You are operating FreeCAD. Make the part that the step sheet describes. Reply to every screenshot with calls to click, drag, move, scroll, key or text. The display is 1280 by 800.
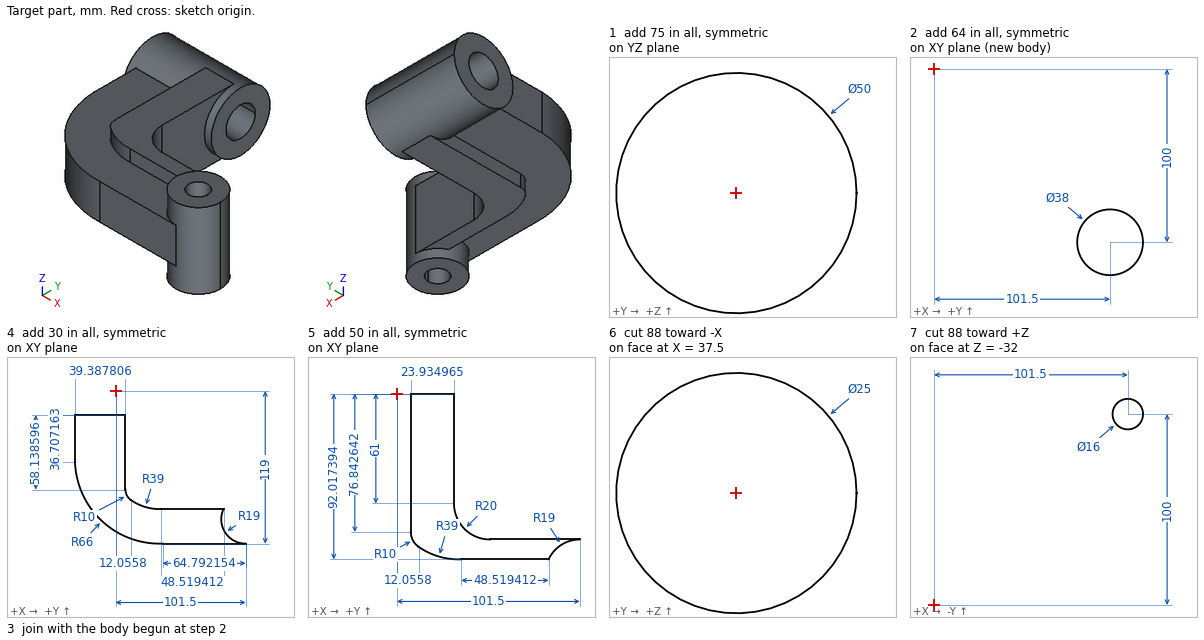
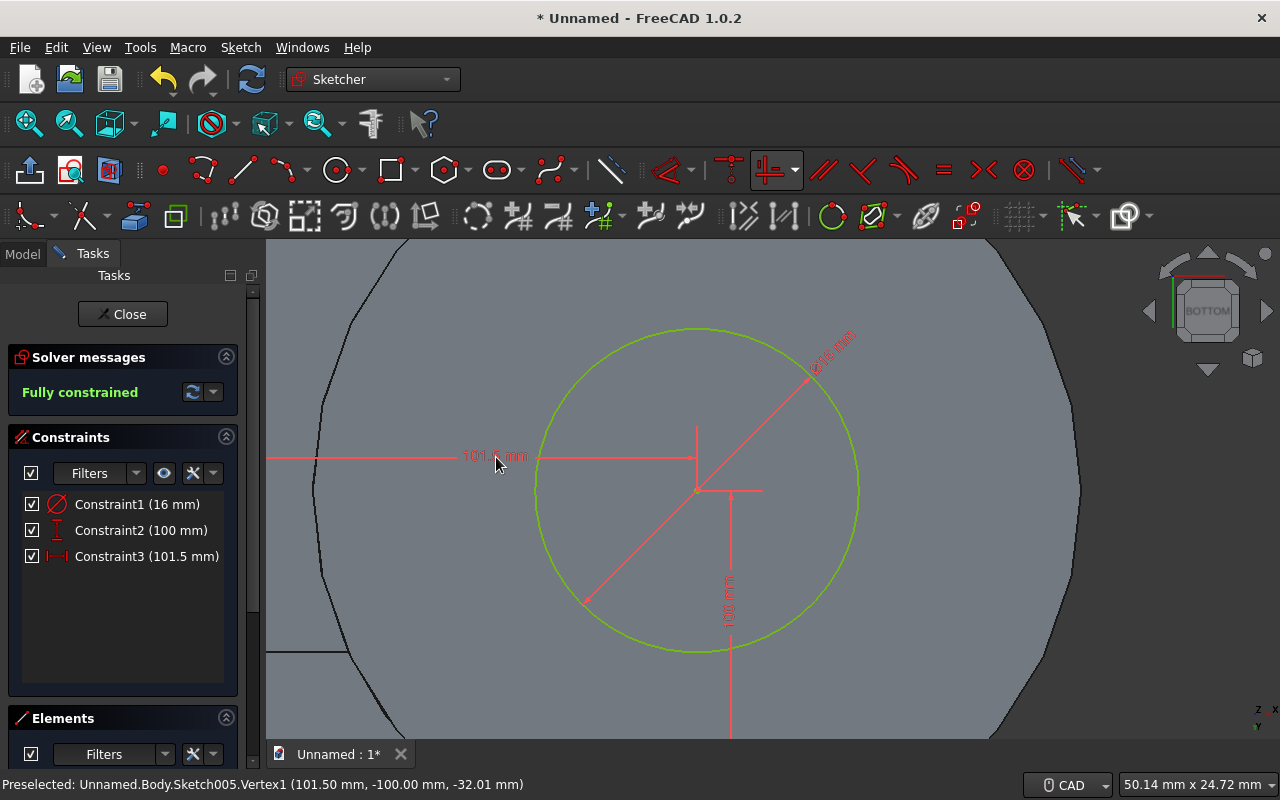
click(123, 314)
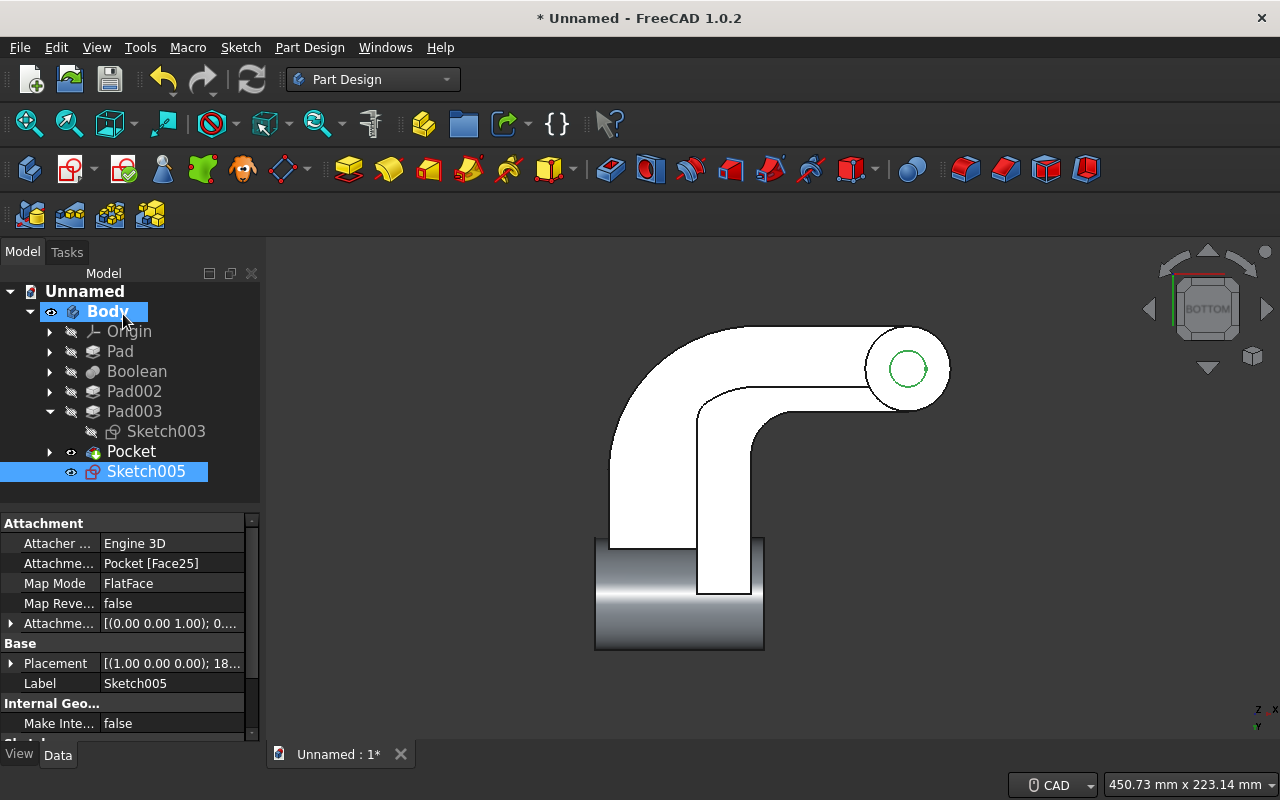
click(612, 170)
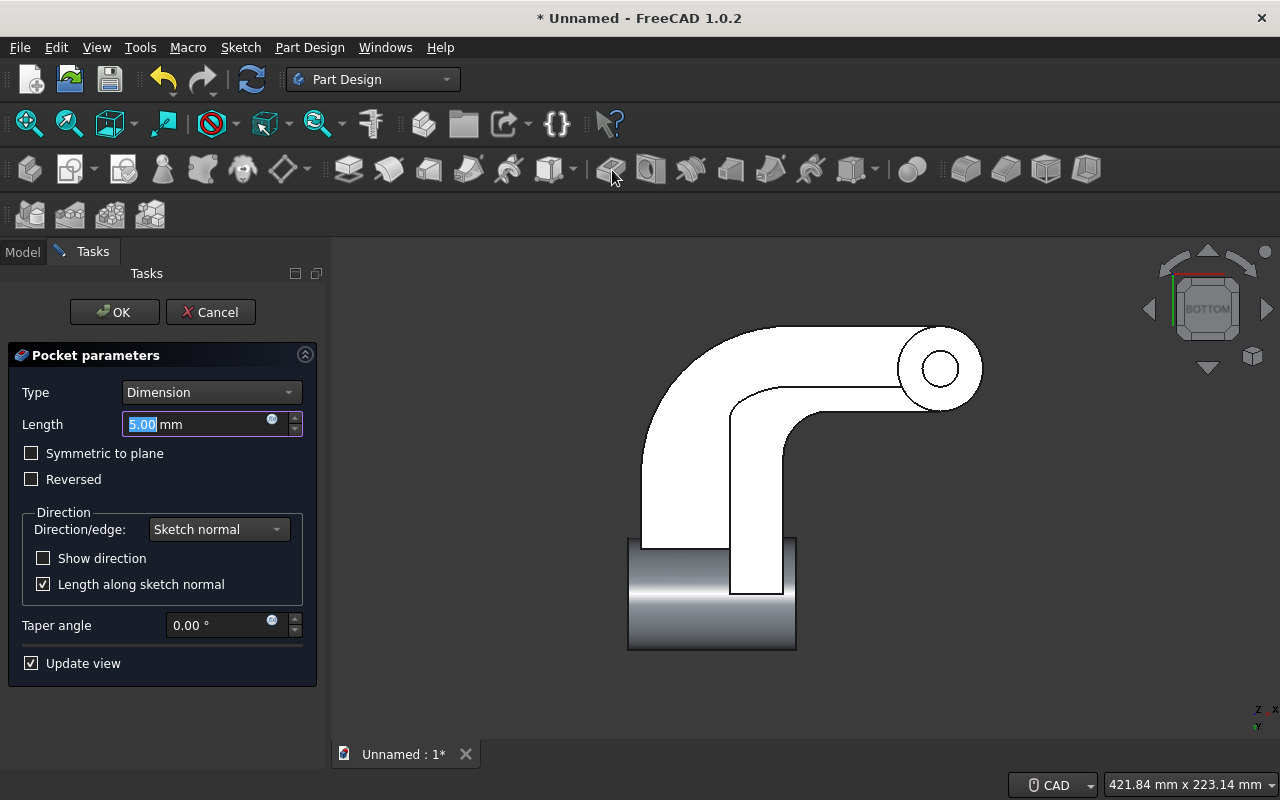
text(88)
key(Tab)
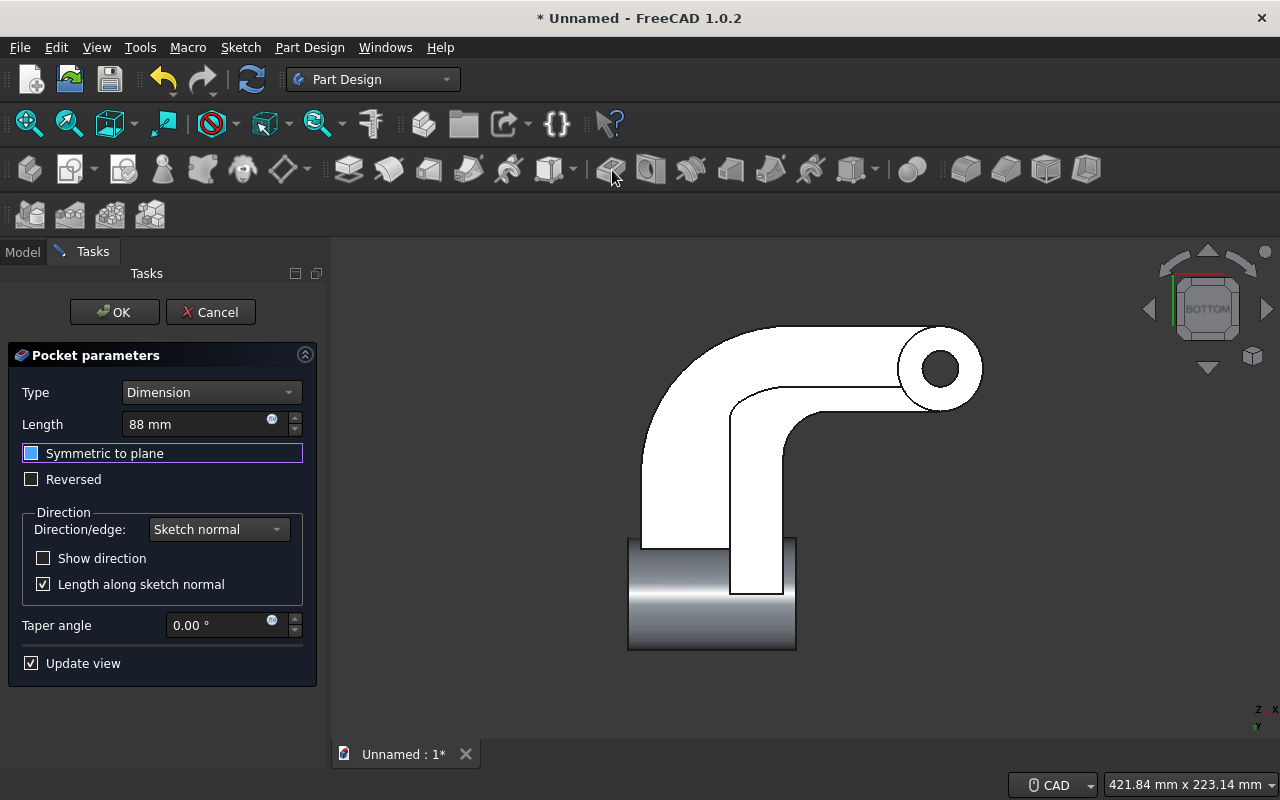
click(115, 312)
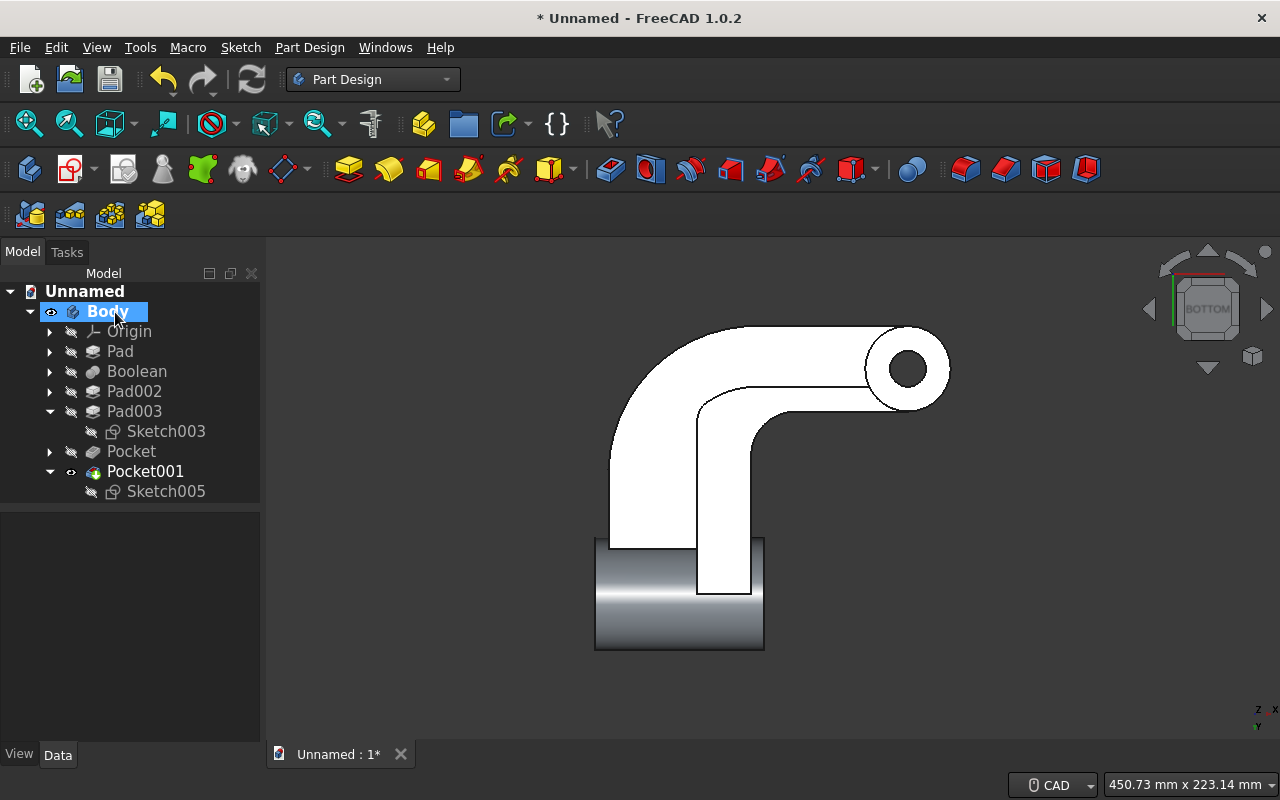
key(0)